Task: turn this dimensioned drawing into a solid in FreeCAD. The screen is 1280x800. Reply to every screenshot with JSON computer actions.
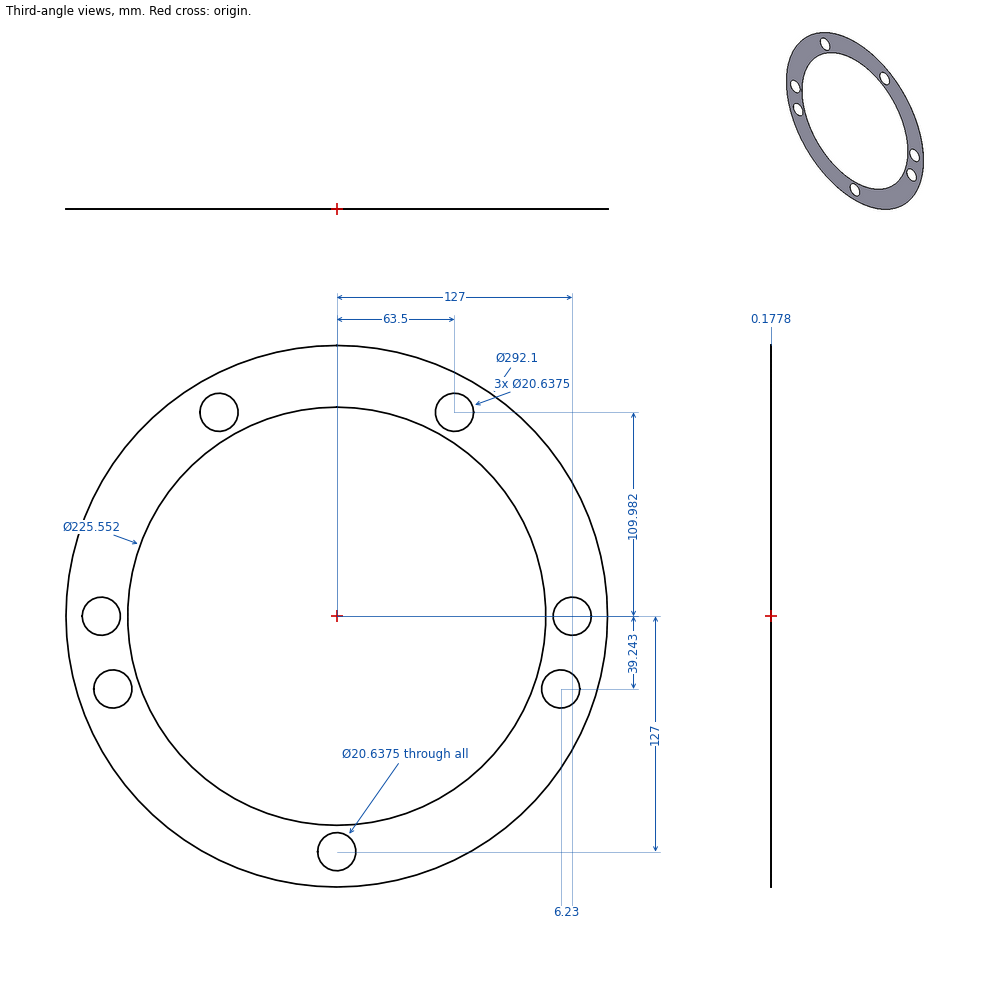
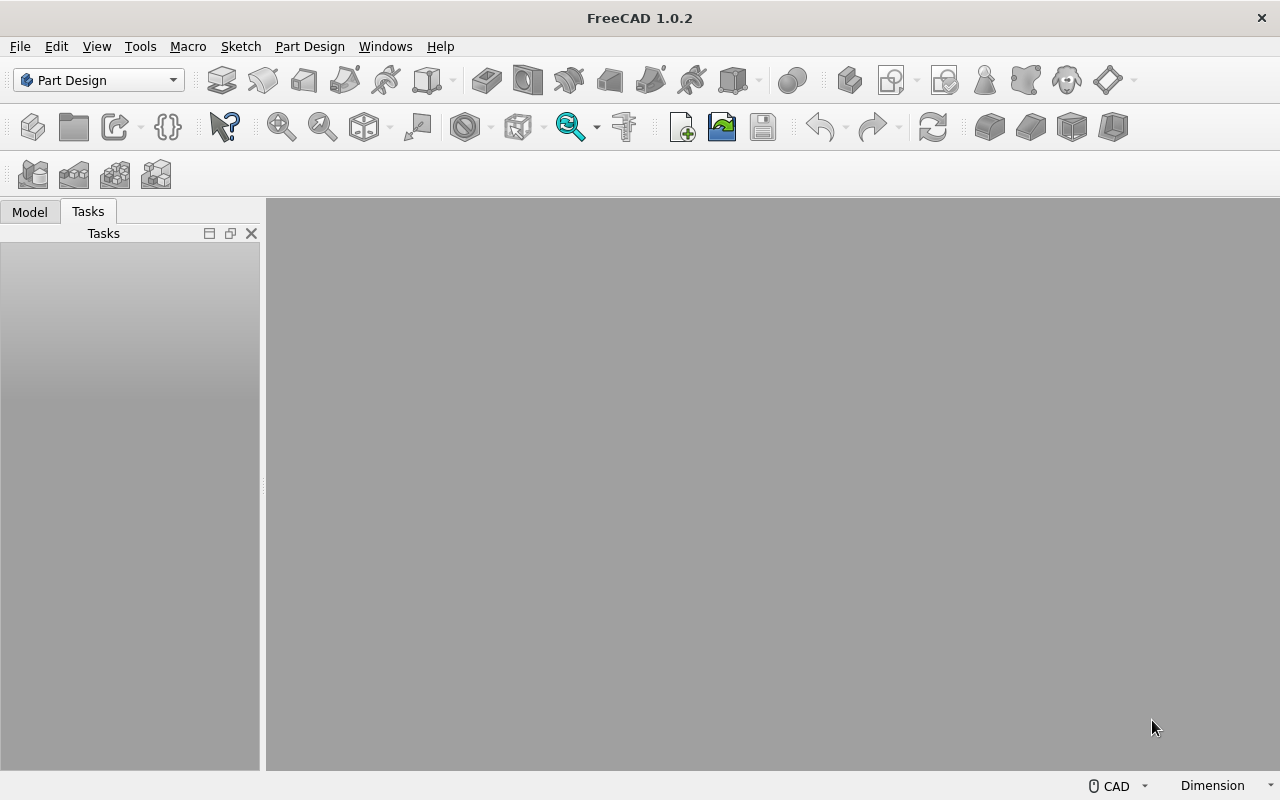
{"action": "key", "text": "ctrl+n"}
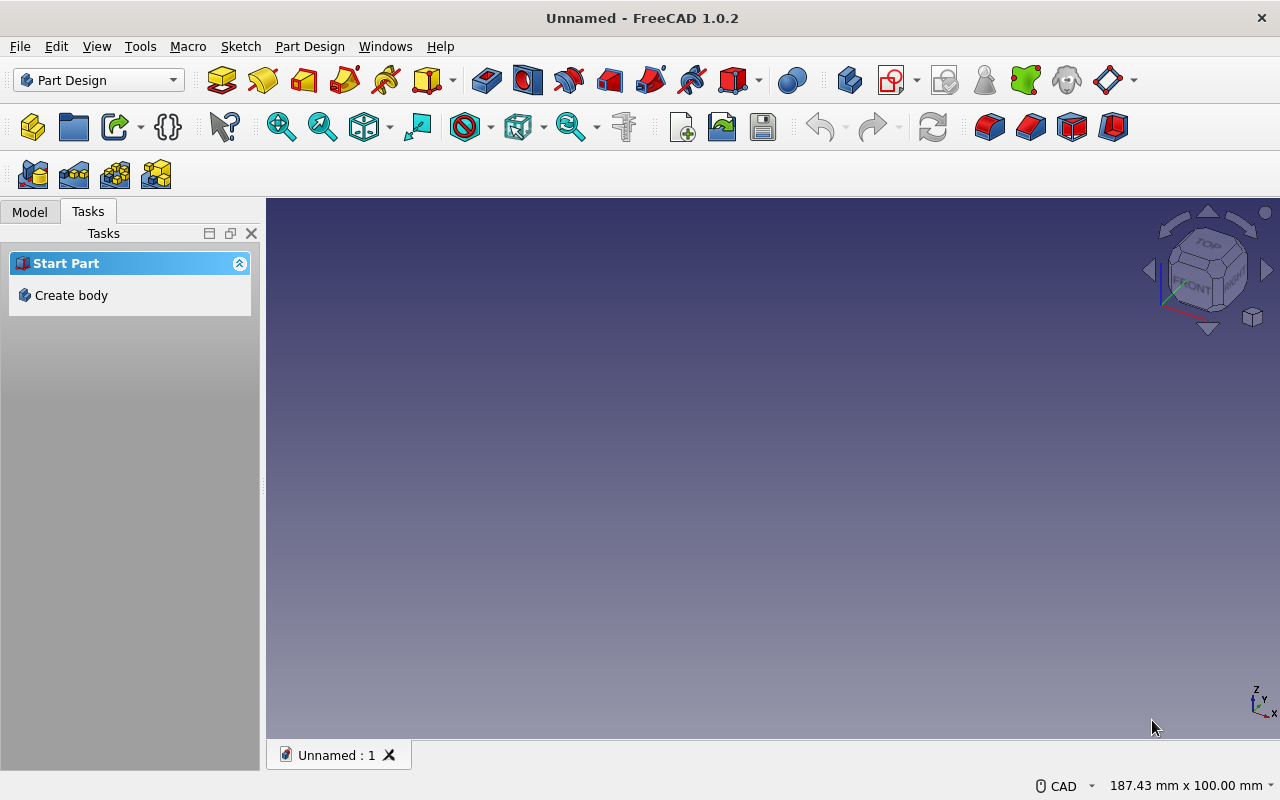
{"action": "left_click", "coordinate": [890, 80]}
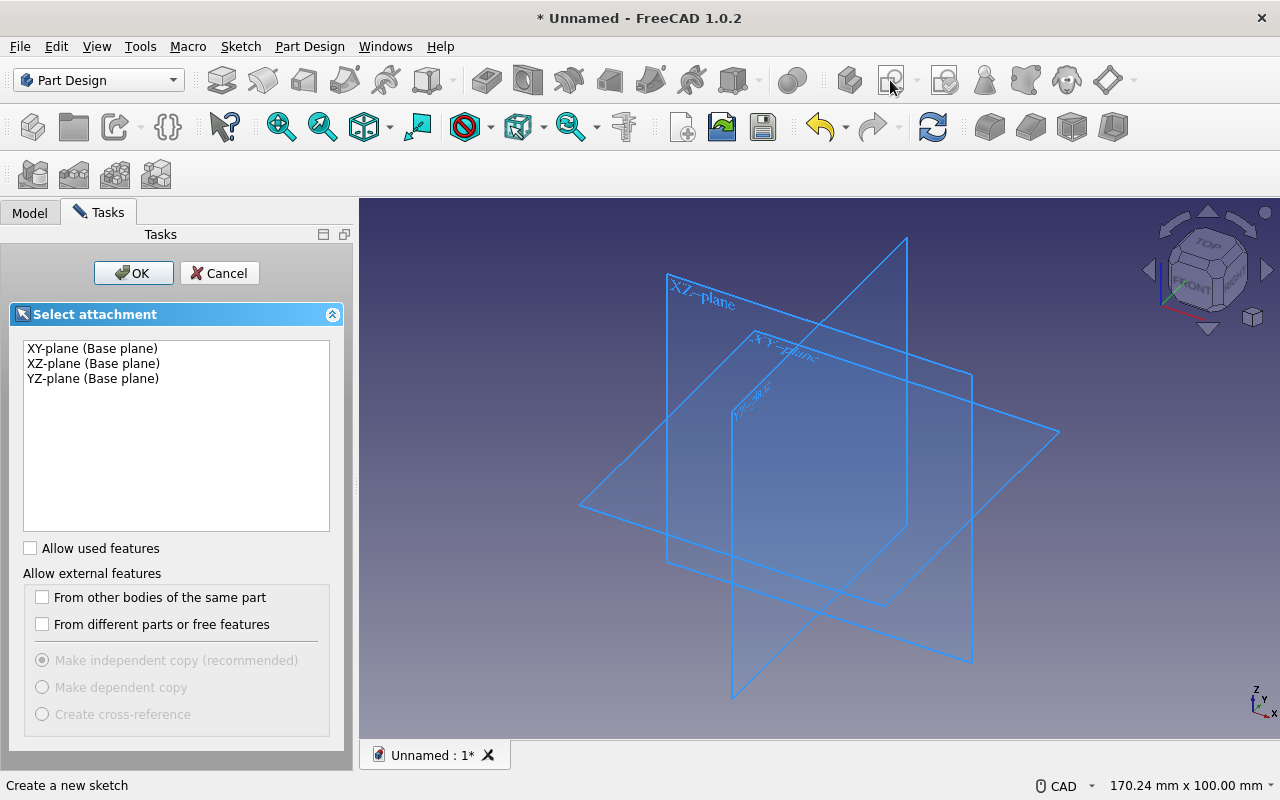
{"action": "left_click", "coordinate": [84, 364]}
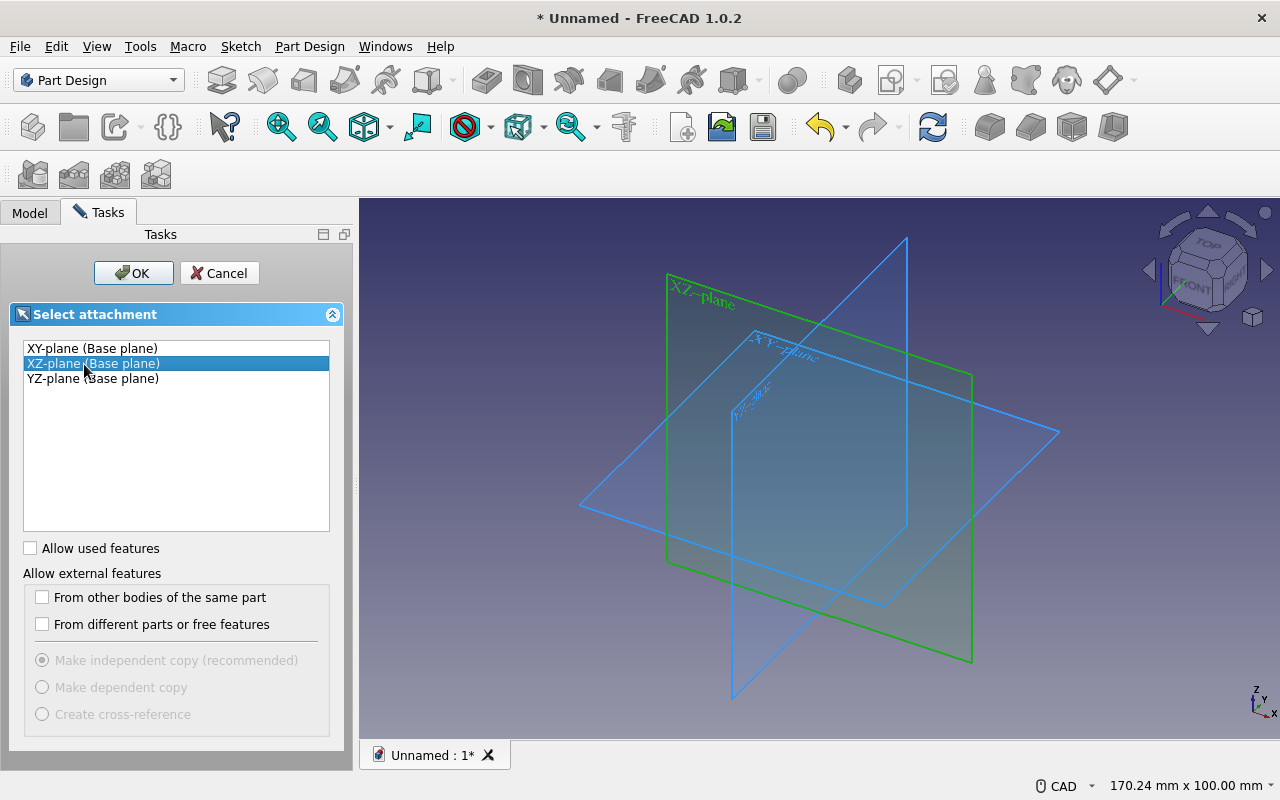
{"action": "left_click", "coordinate": [134, 273]}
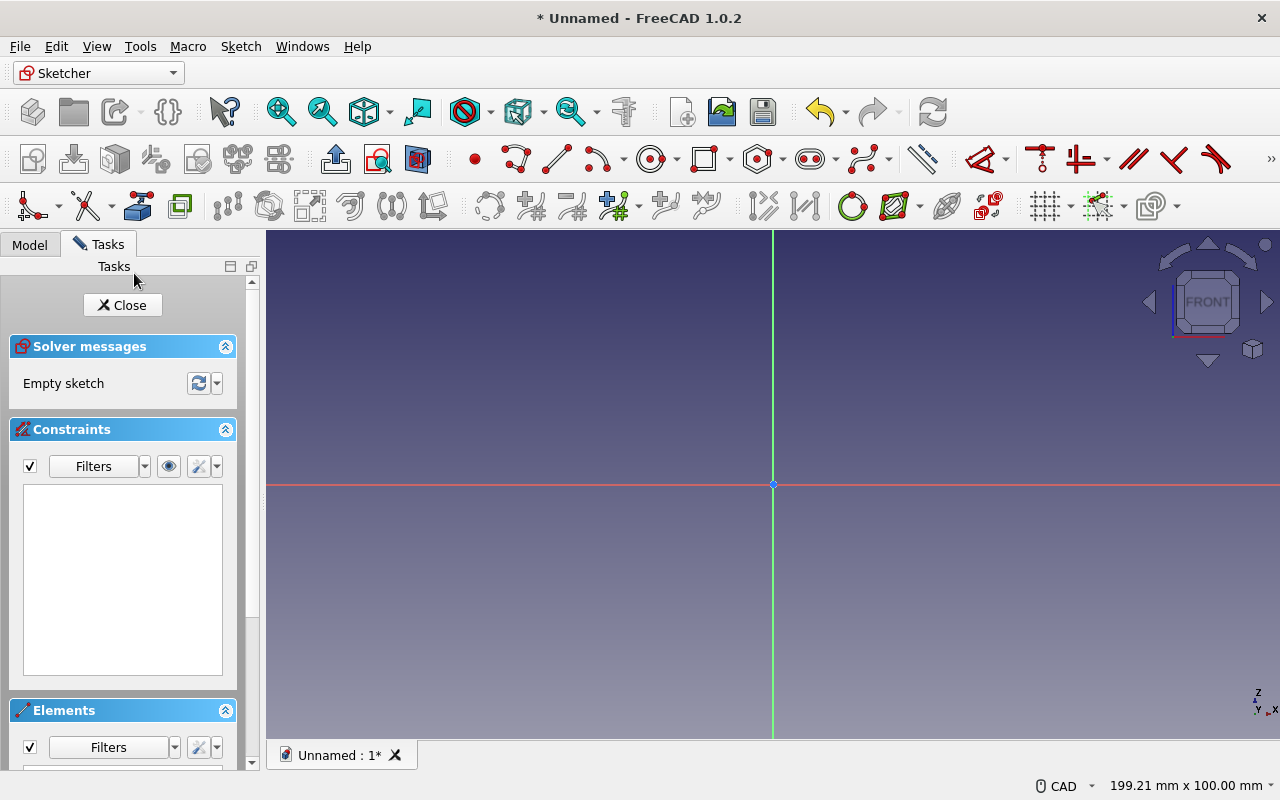
{"action": "scroll", "coordinate": [687, 484], "scroll_direction": "down", "scroll_amount": 8}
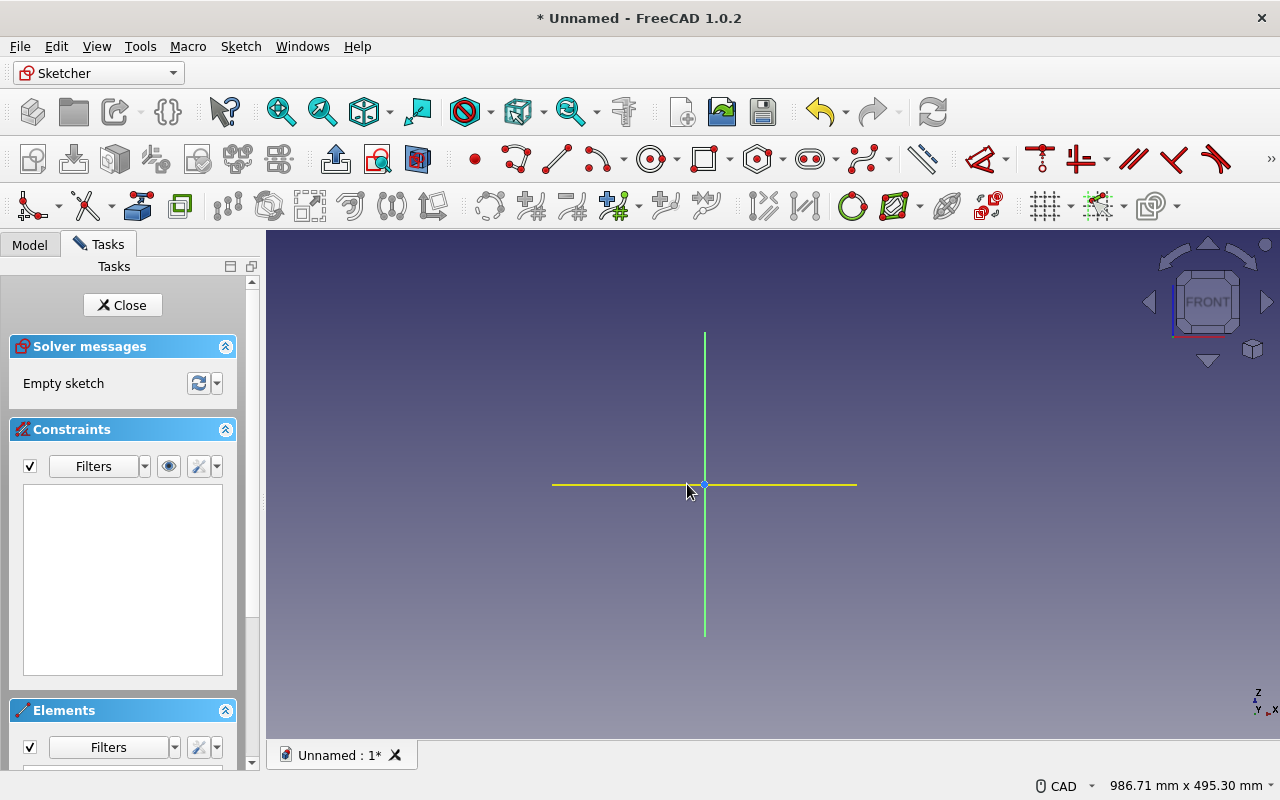
{"action": "key", "text": "g c"}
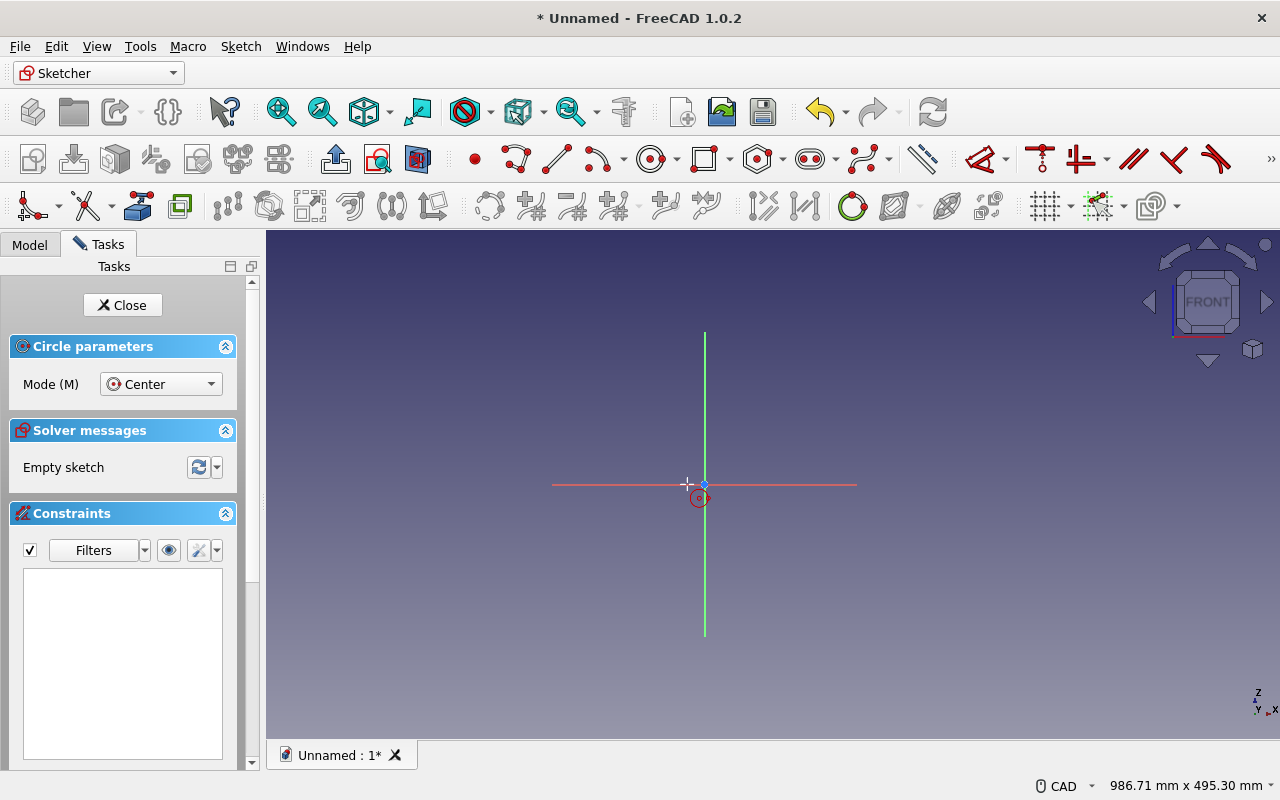
{"action": "left_click", "coordinate": [705, 484]}
{"action": "mouse_move", "coordinate": [811, 378]}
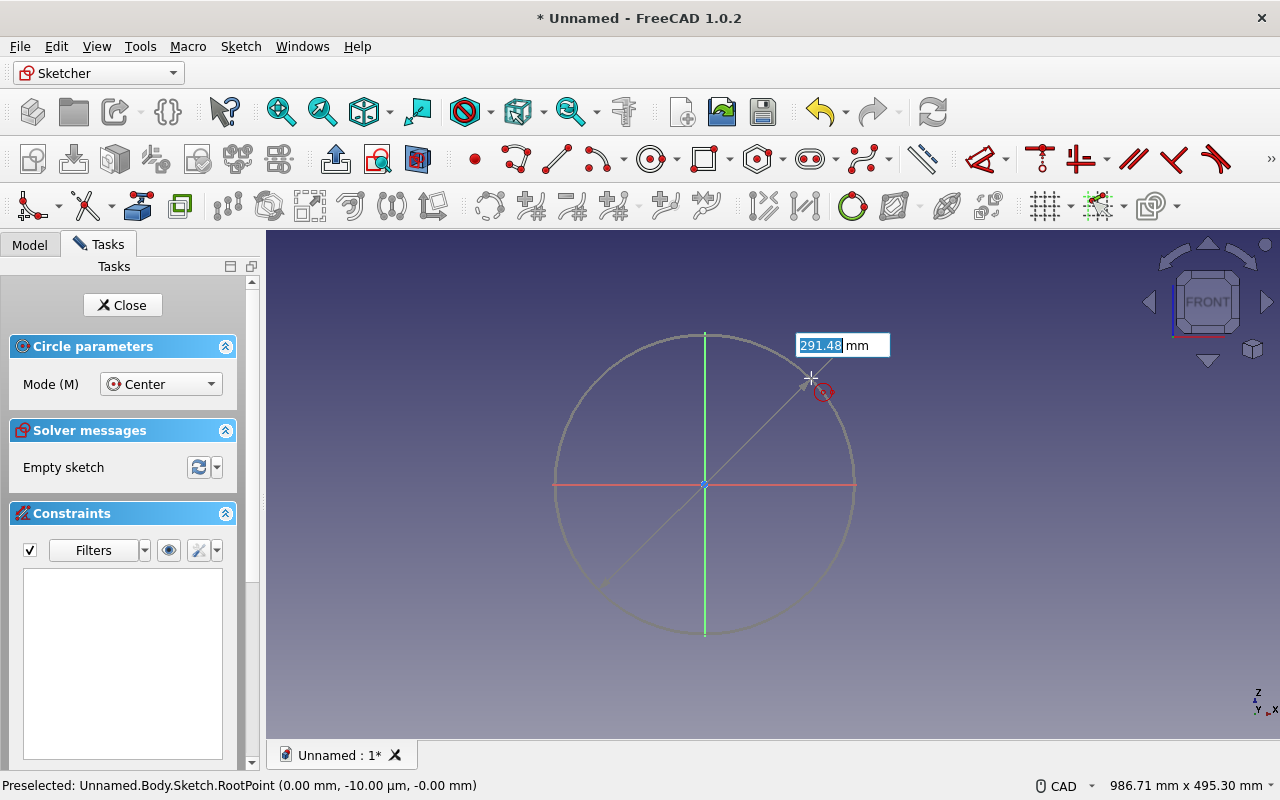
{"action": "type", "text": "292.1"}
{"action": "key", "text": "Return"}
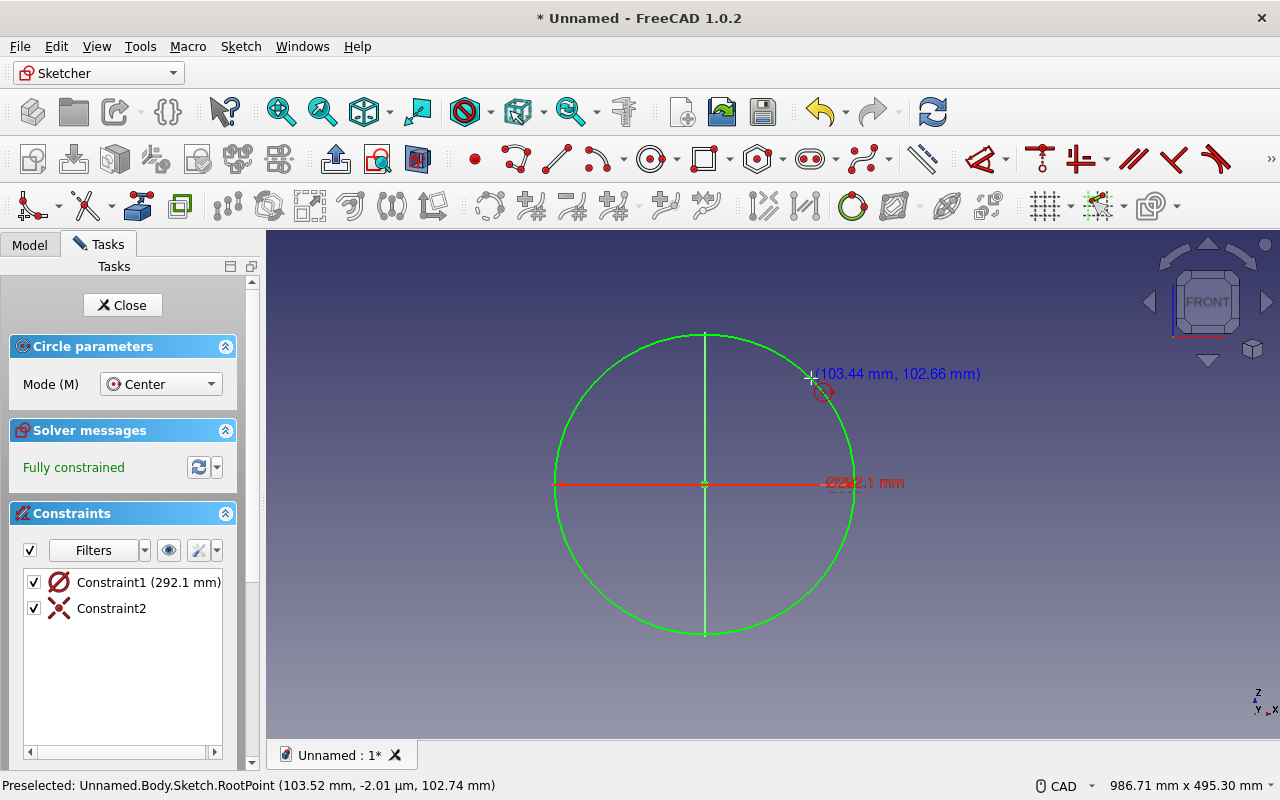
{"action": "left_click", "coordinate": [705, 484]}
{"action": "mouse_move", "coordinate": [787, 403]}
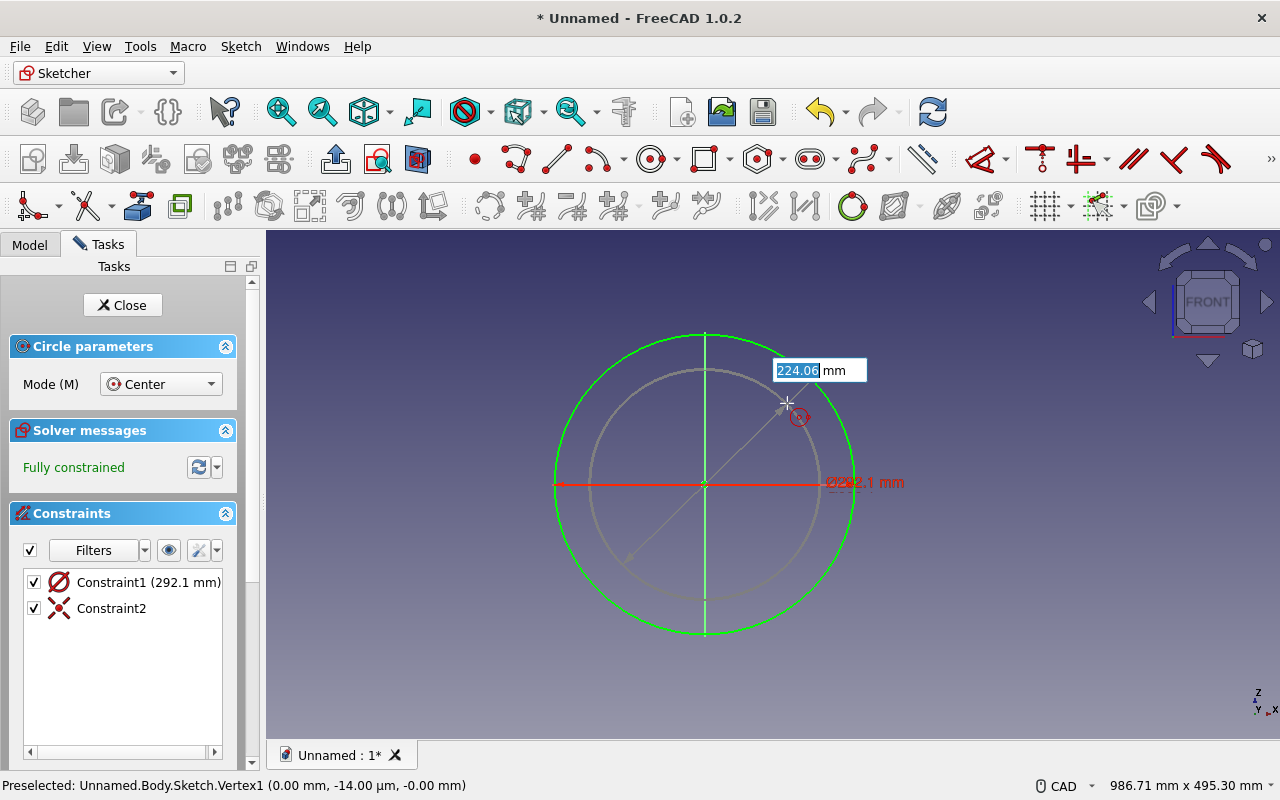
{"action": "type", "text": "225.552"}
{"action": "key", "text": "Return"}
{"action": "key", "text": "Escape"}